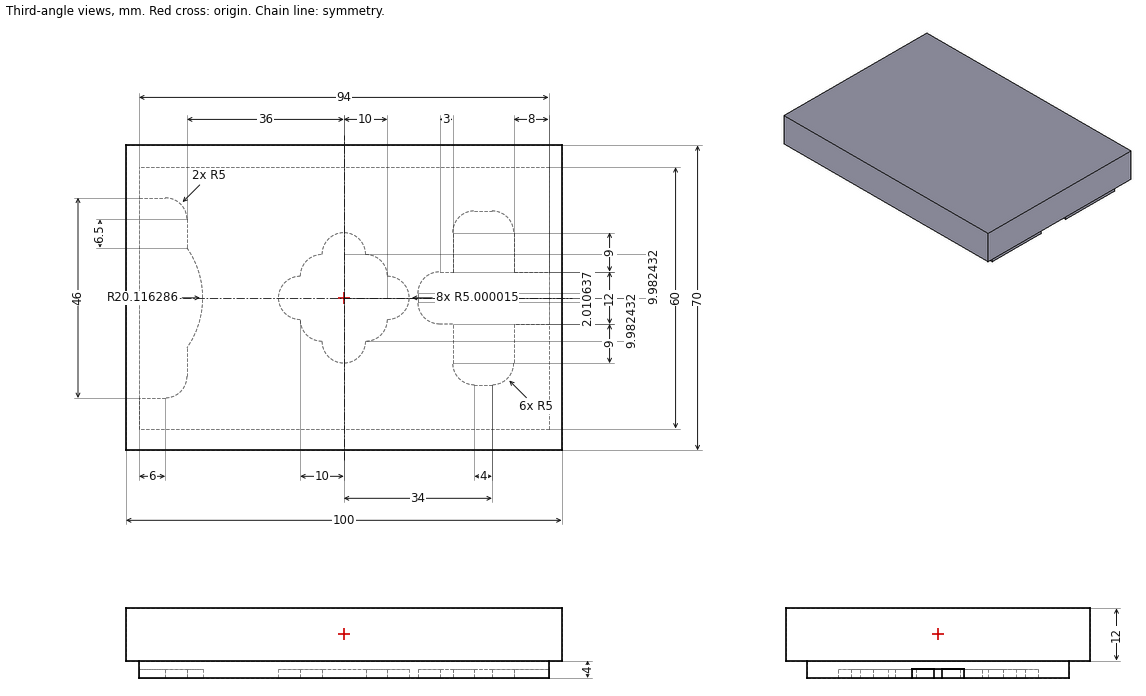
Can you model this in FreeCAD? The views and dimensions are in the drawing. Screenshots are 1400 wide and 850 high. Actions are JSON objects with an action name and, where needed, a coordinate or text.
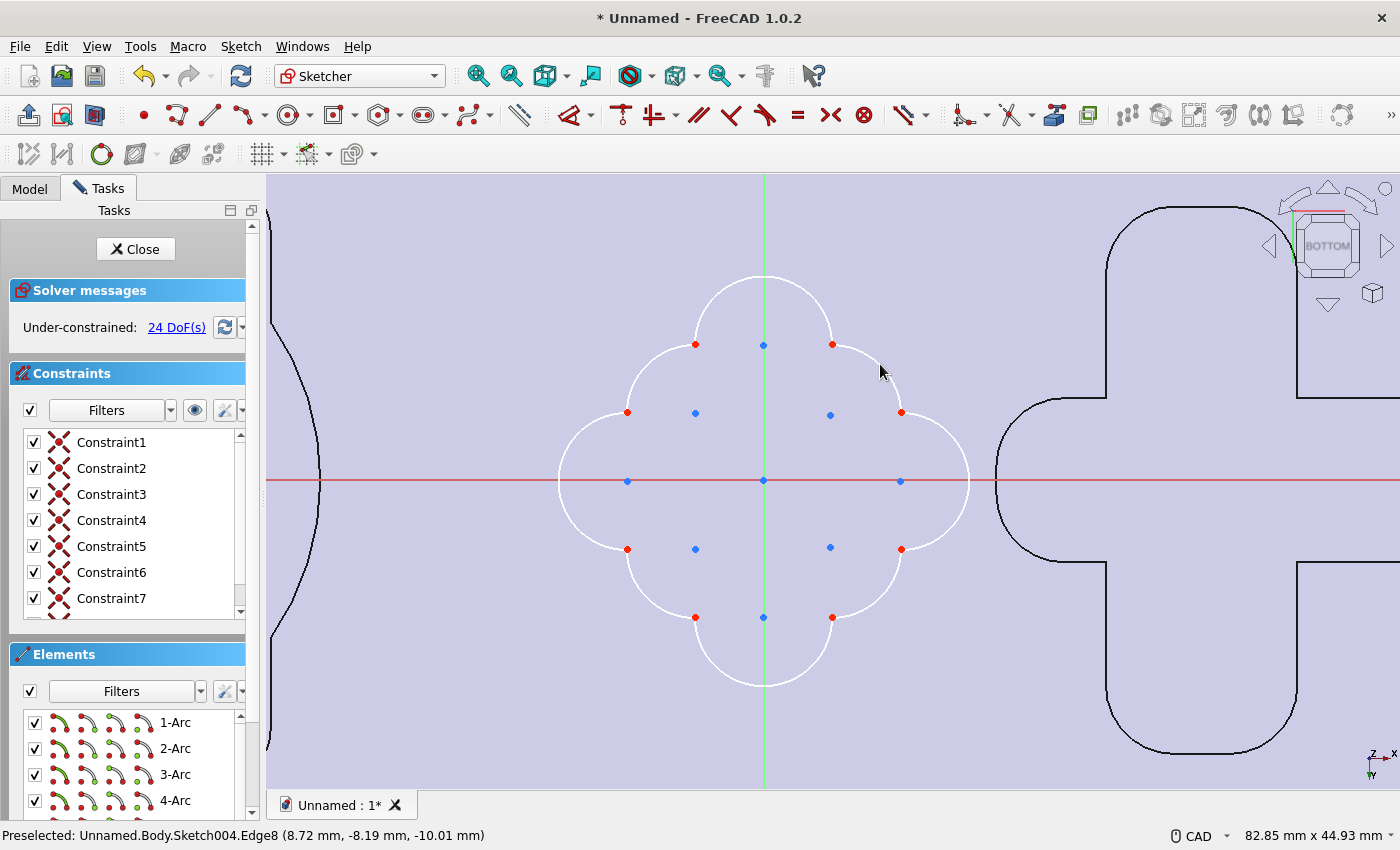
{"action": "left_click", "coordinate": [804, 290]}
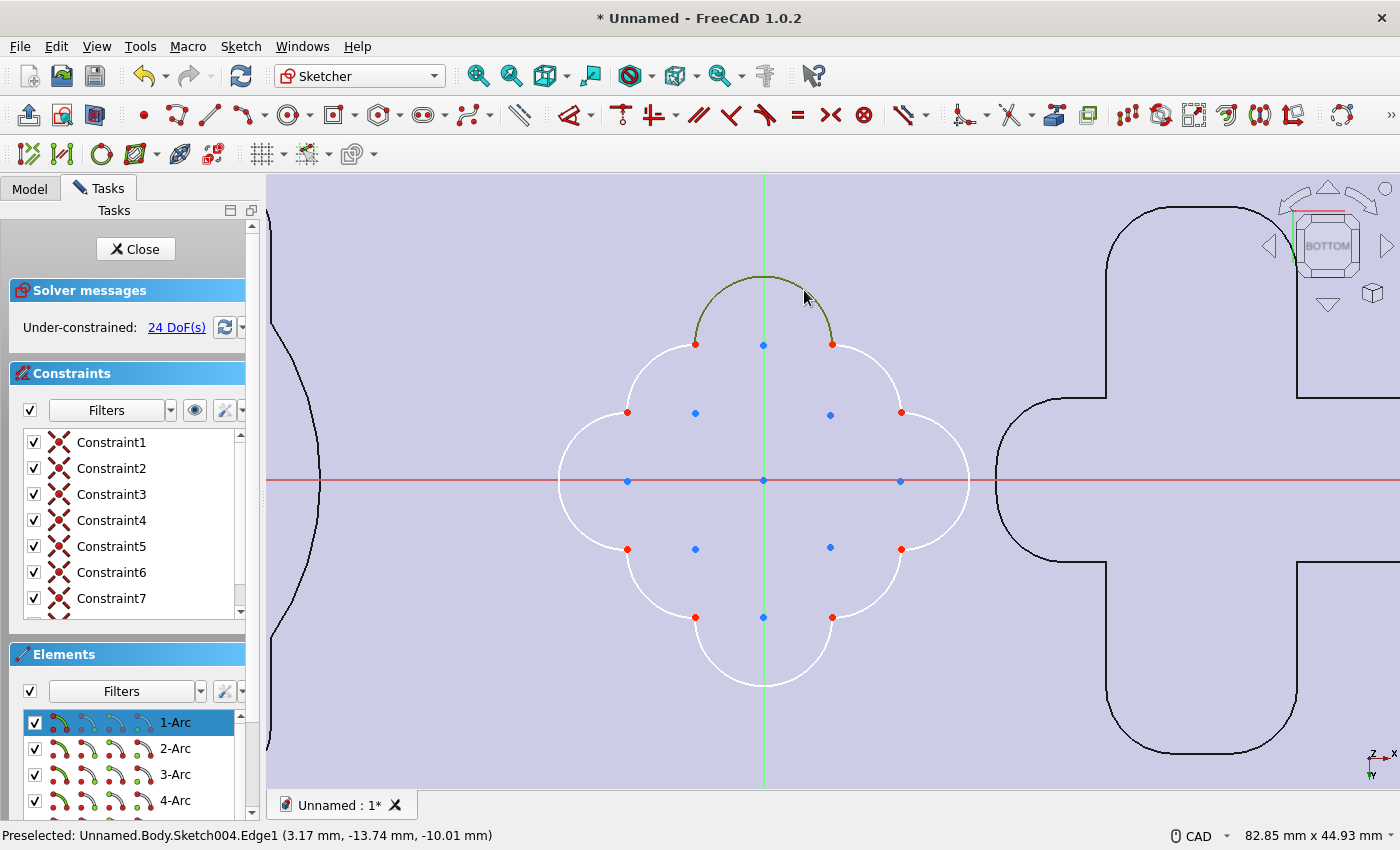
{"action": "left_click", "coordinate": [664, 352]}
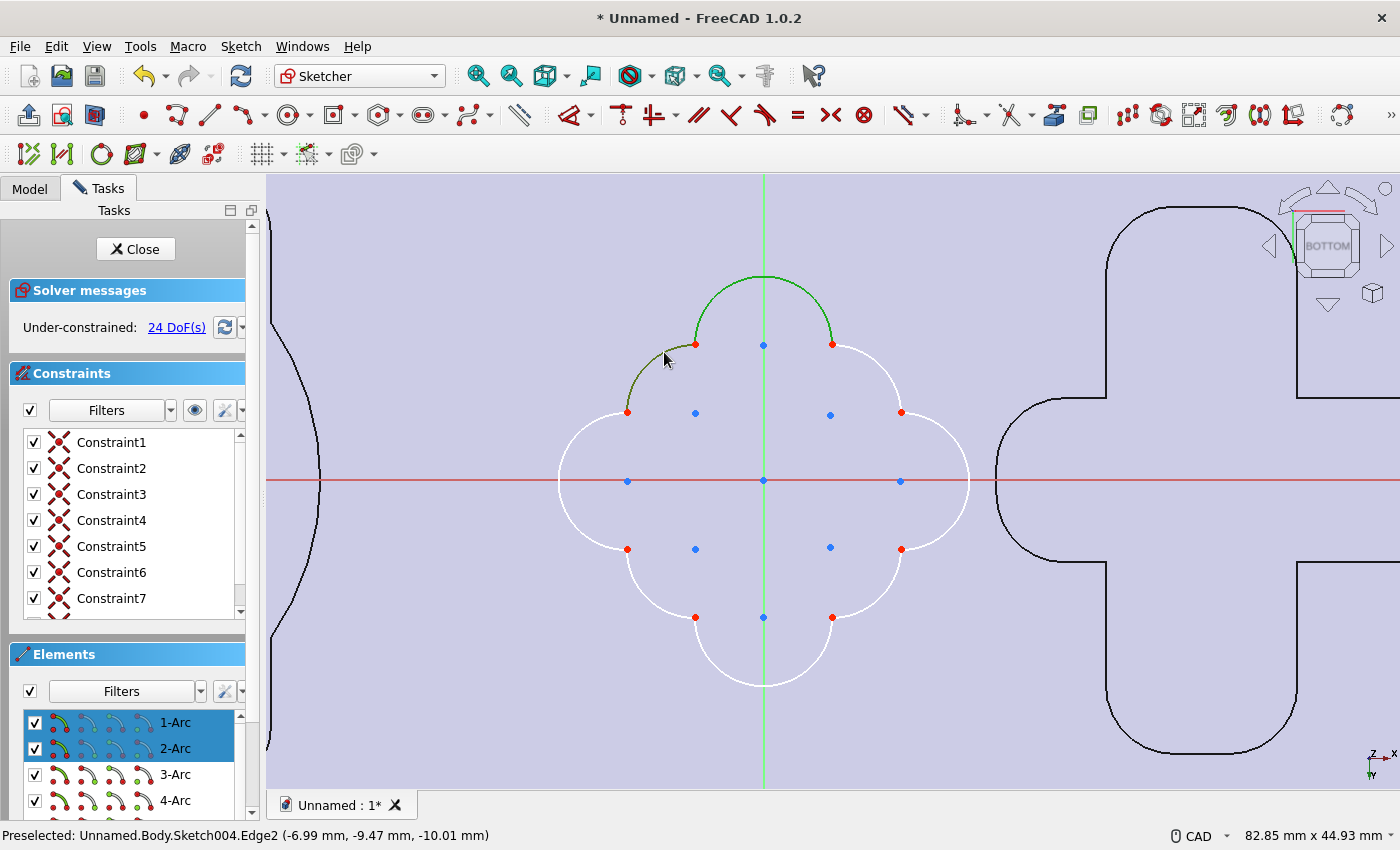
{"action": "left_click", "coordinate": [572, 441]}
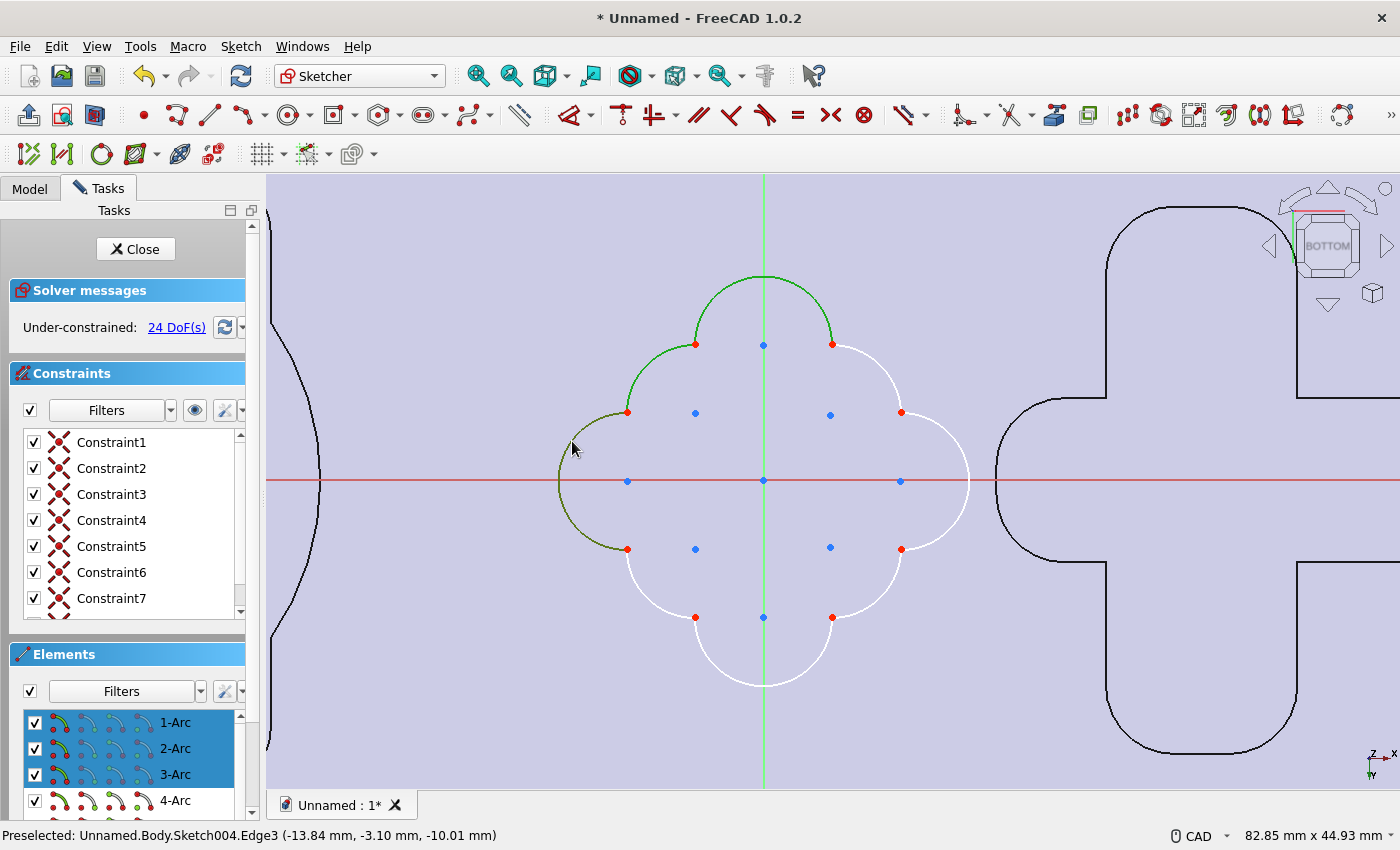
{"action": "left_click", "coordinate": [634, 581]}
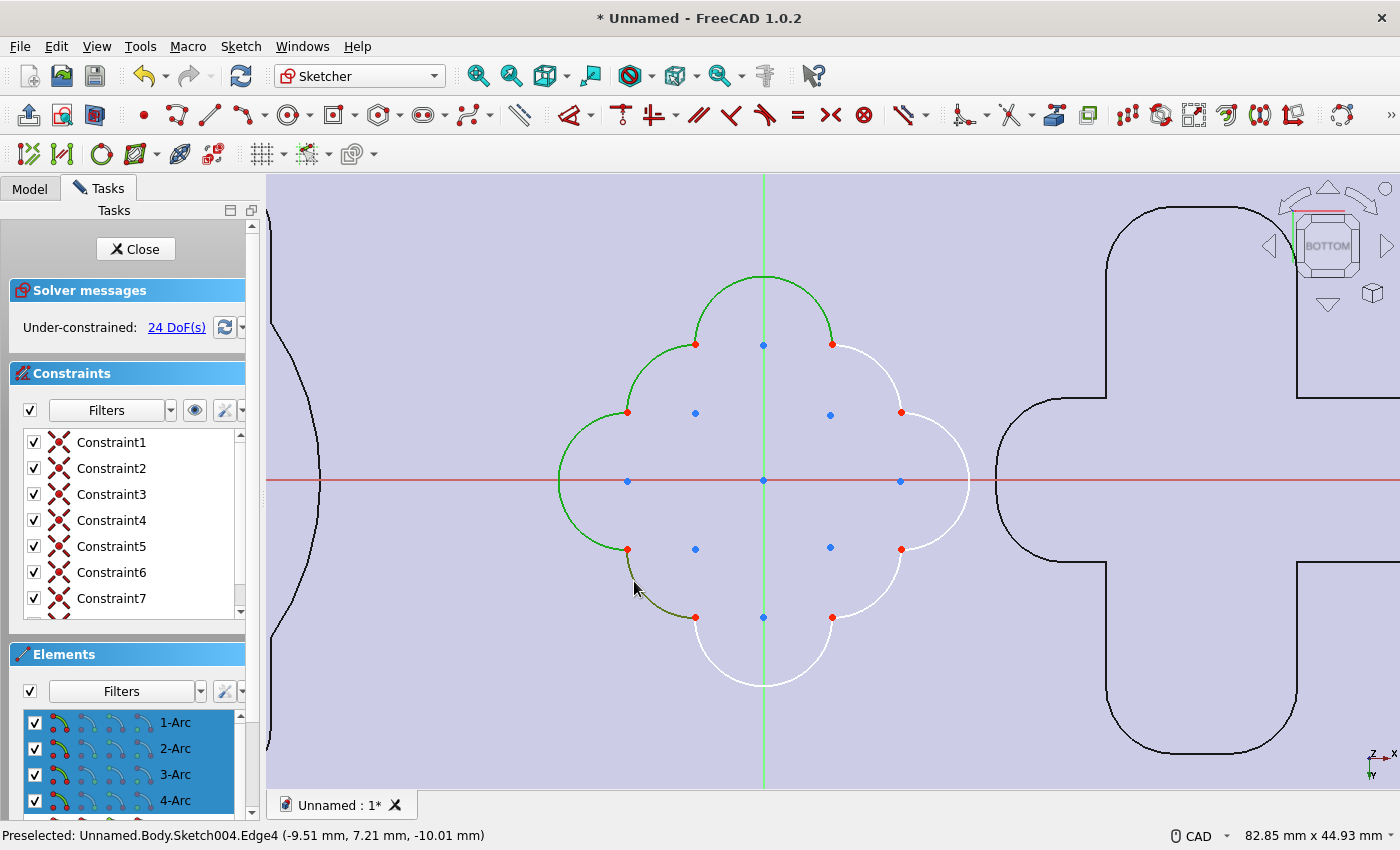
{"action": "left_click", "coordinate": [723, 673]}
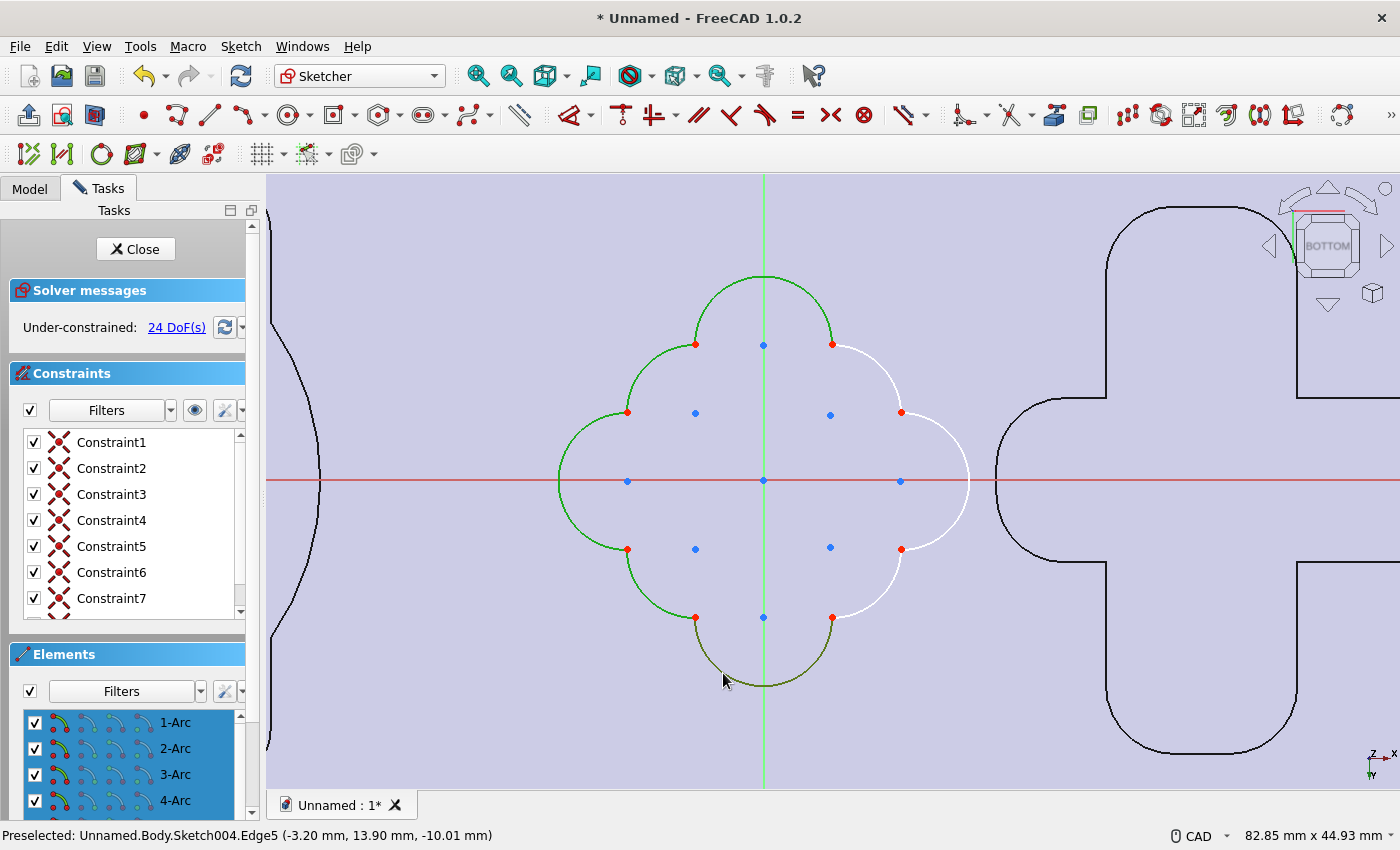
{"action": "left_click", "coordinate": [863, 610]}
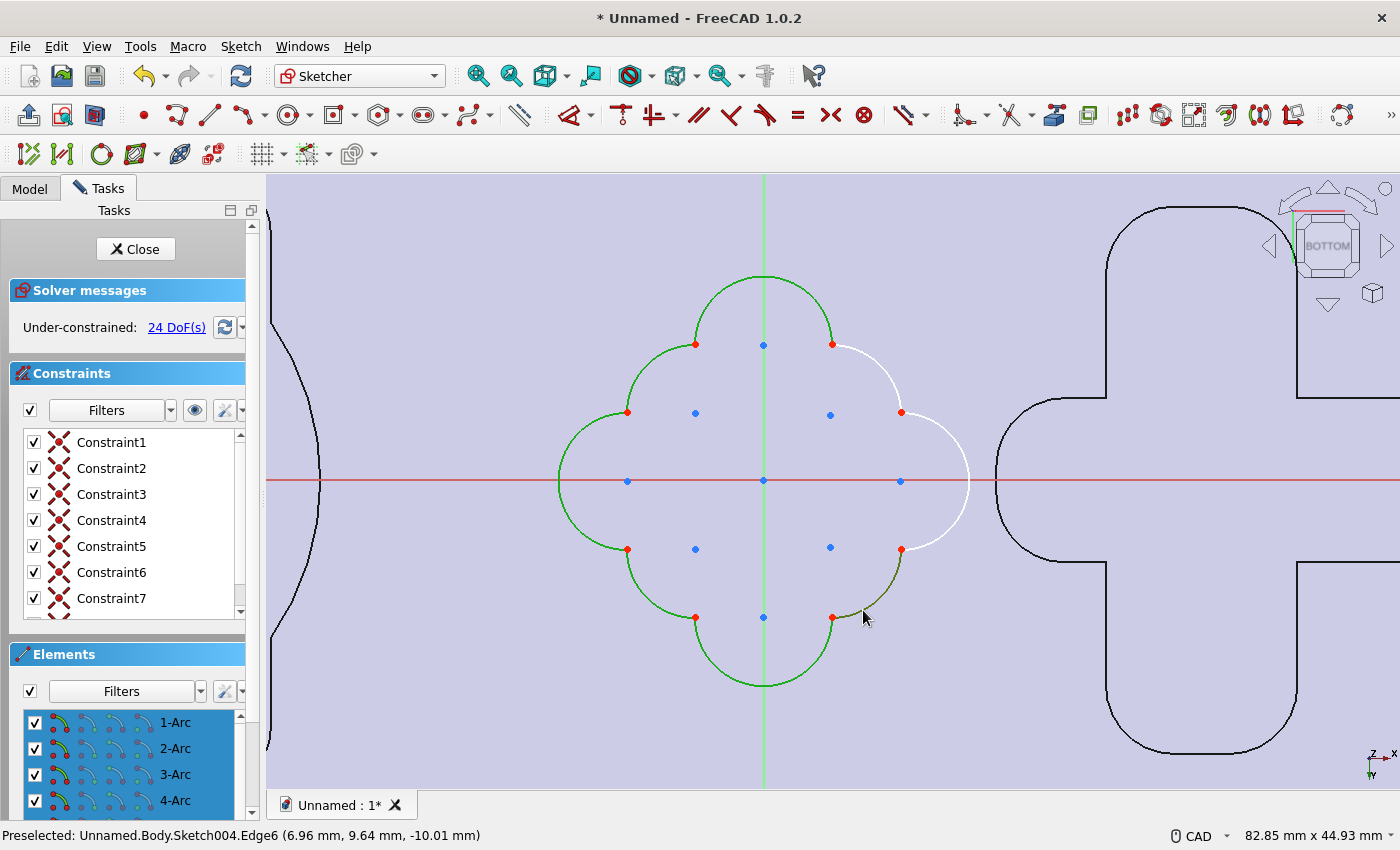
{"action": "left_click", "coordinate": [956, 522]}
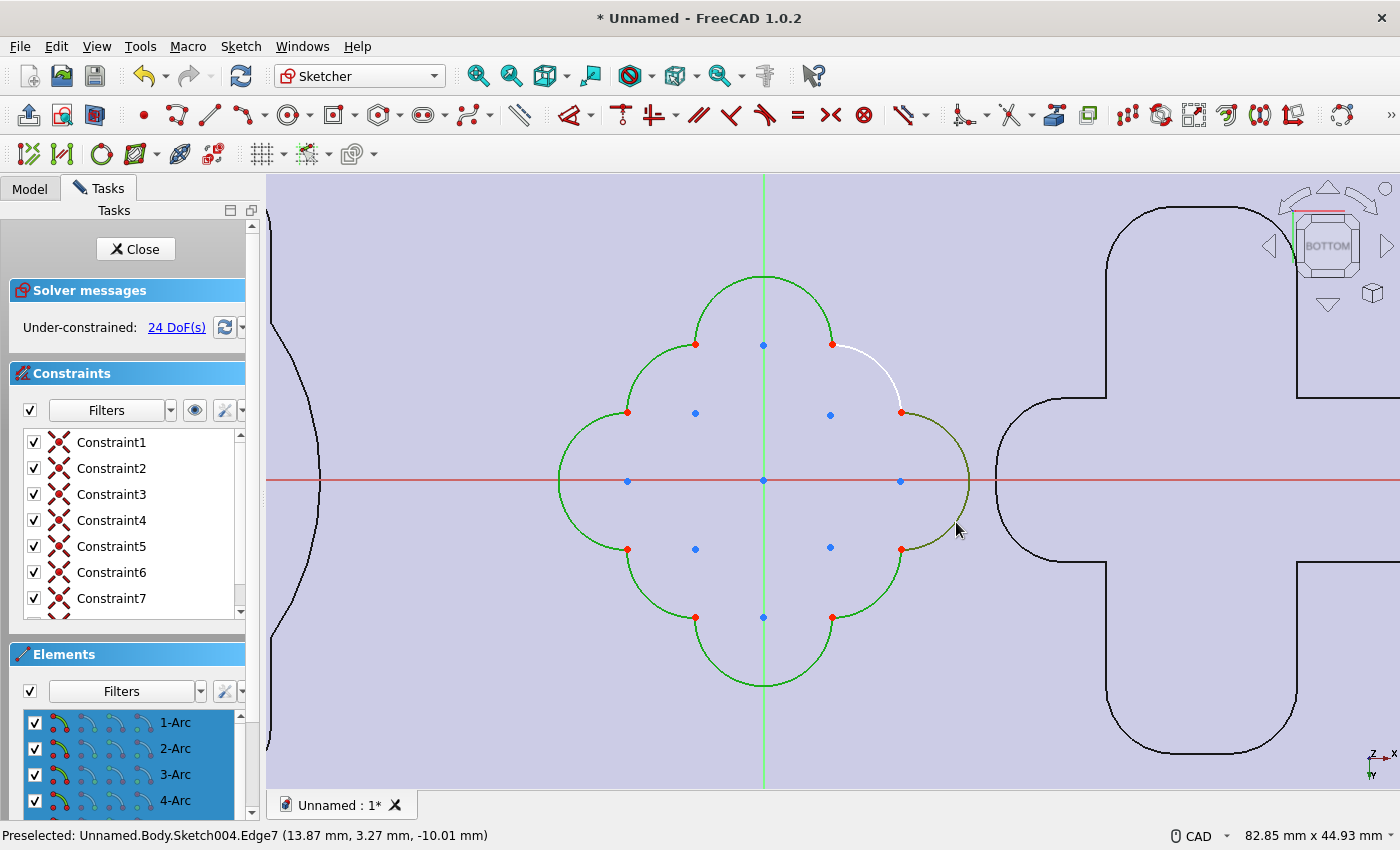
{"action": "left_click", "coordinate": [893, 382]}